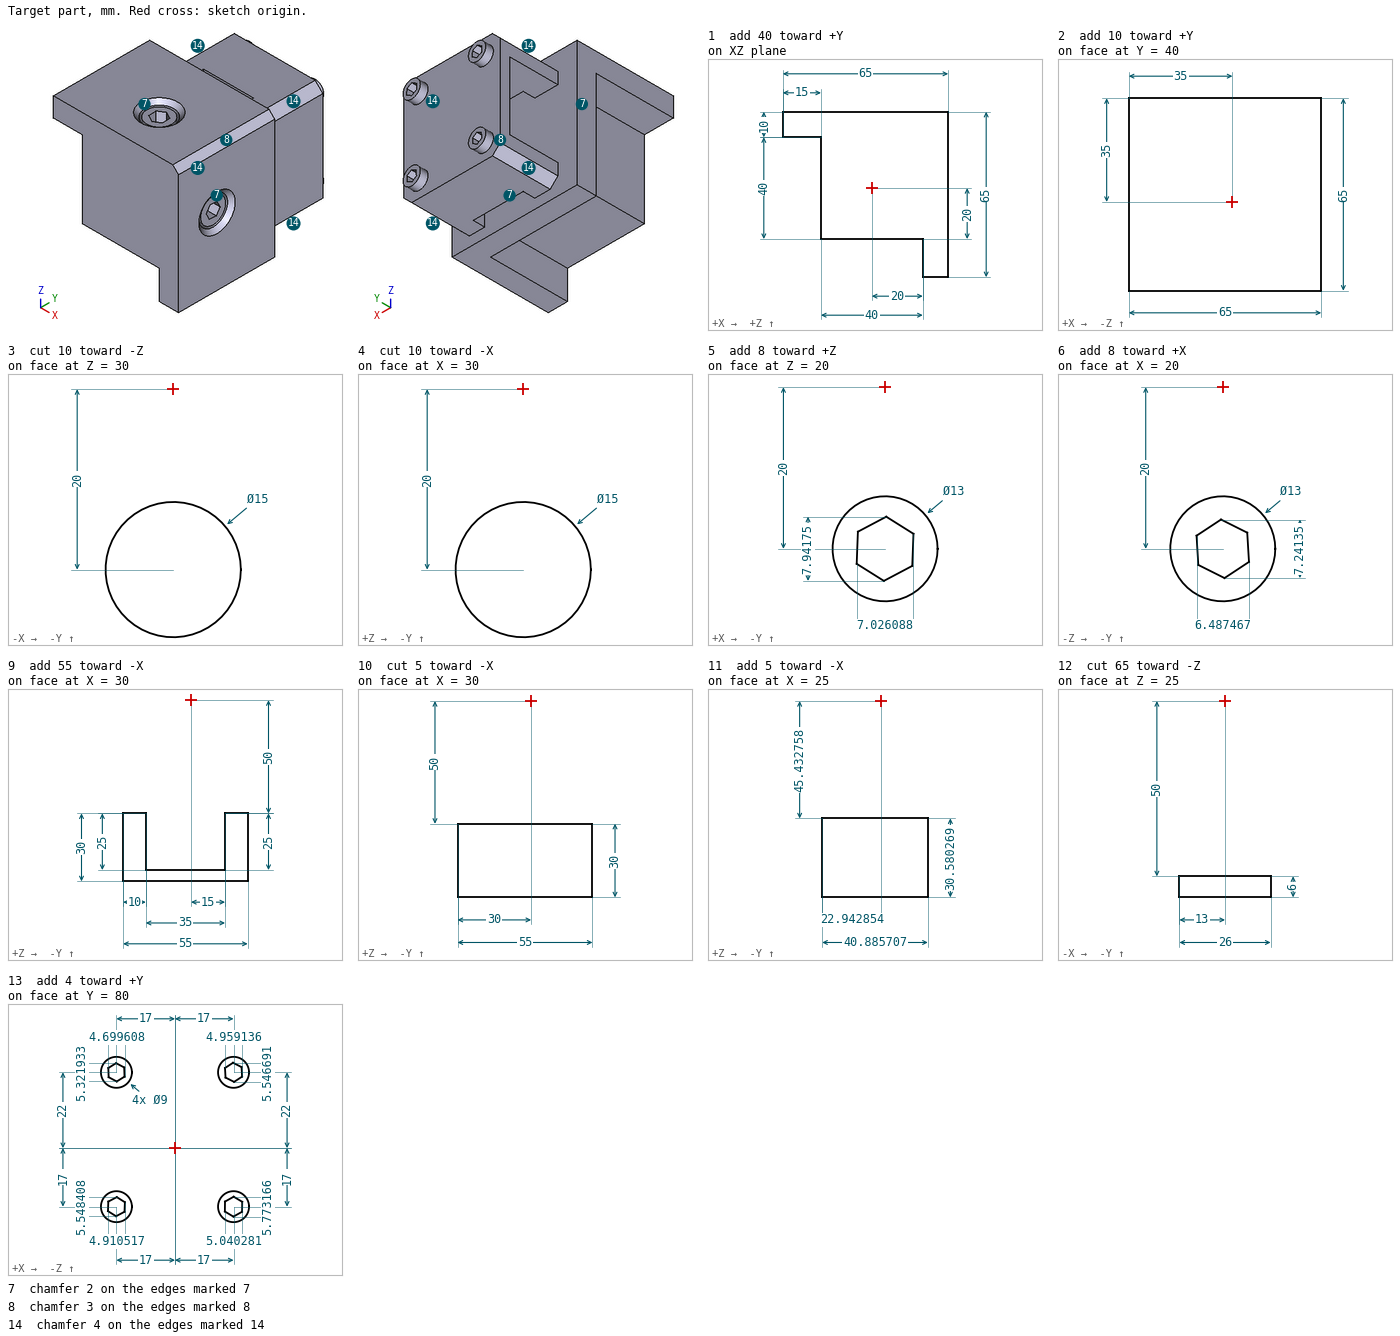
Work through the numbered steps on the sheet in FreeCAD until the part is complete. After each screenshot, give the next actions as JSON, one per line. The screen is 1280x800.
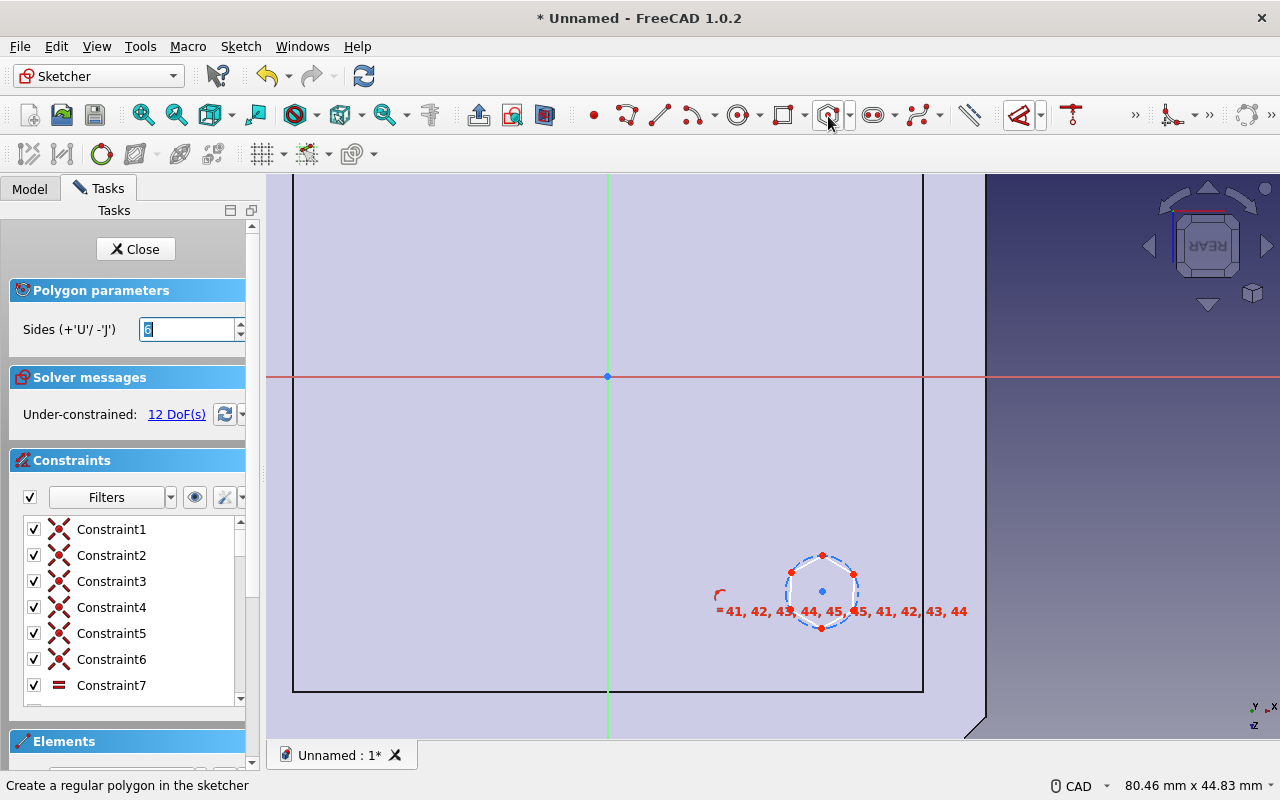
{"action": "left_click", "coordinate": [394, 591]}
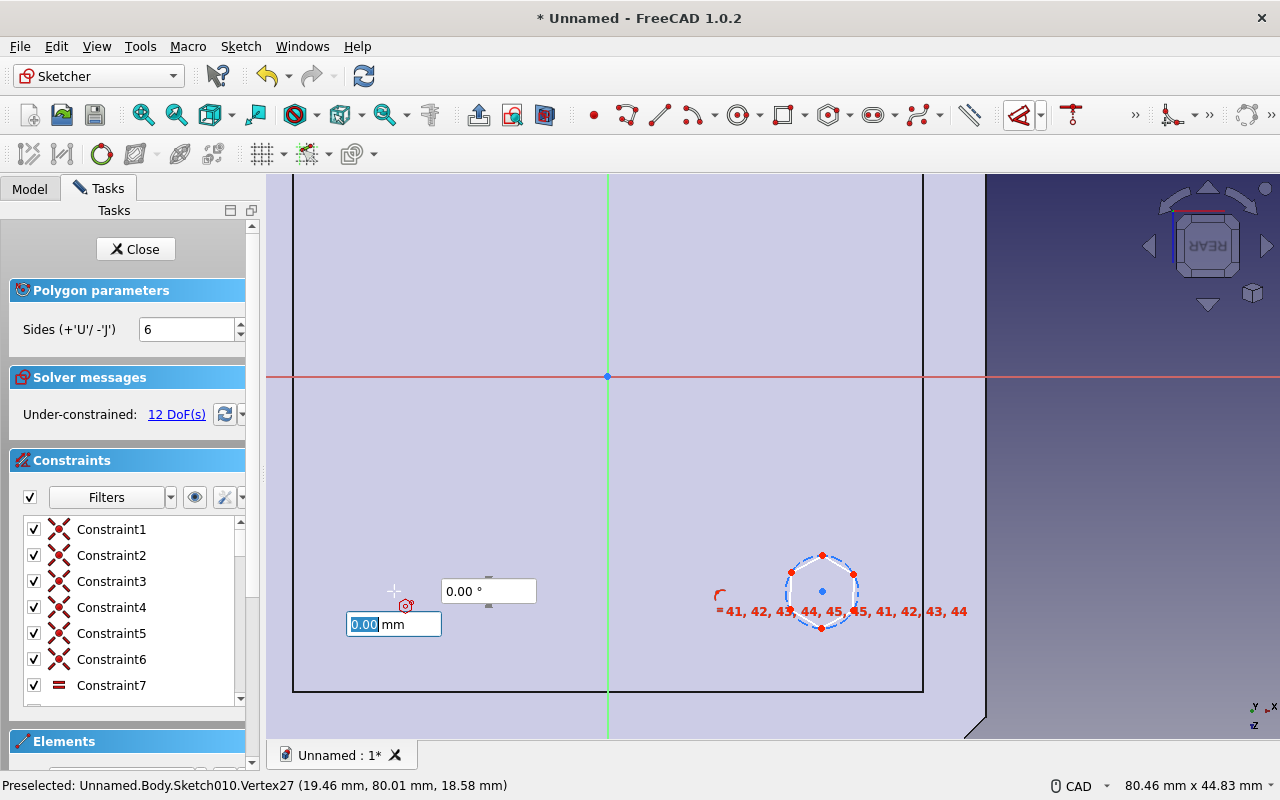
{"action": "left_click", "coordinate": [363, 607]}
{"action": "right_click", "coordinate": [363, 607]}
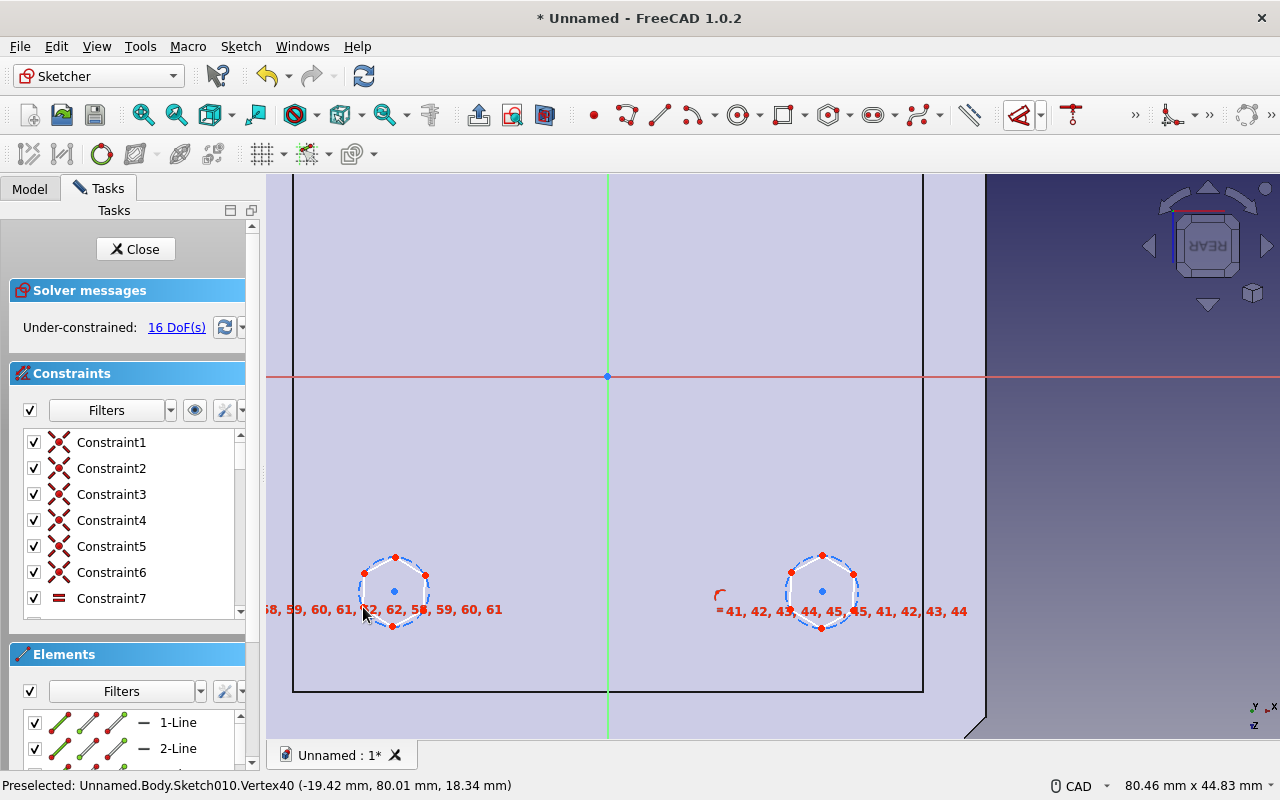
{"action": "left_click", "coordinate": [738, 116]}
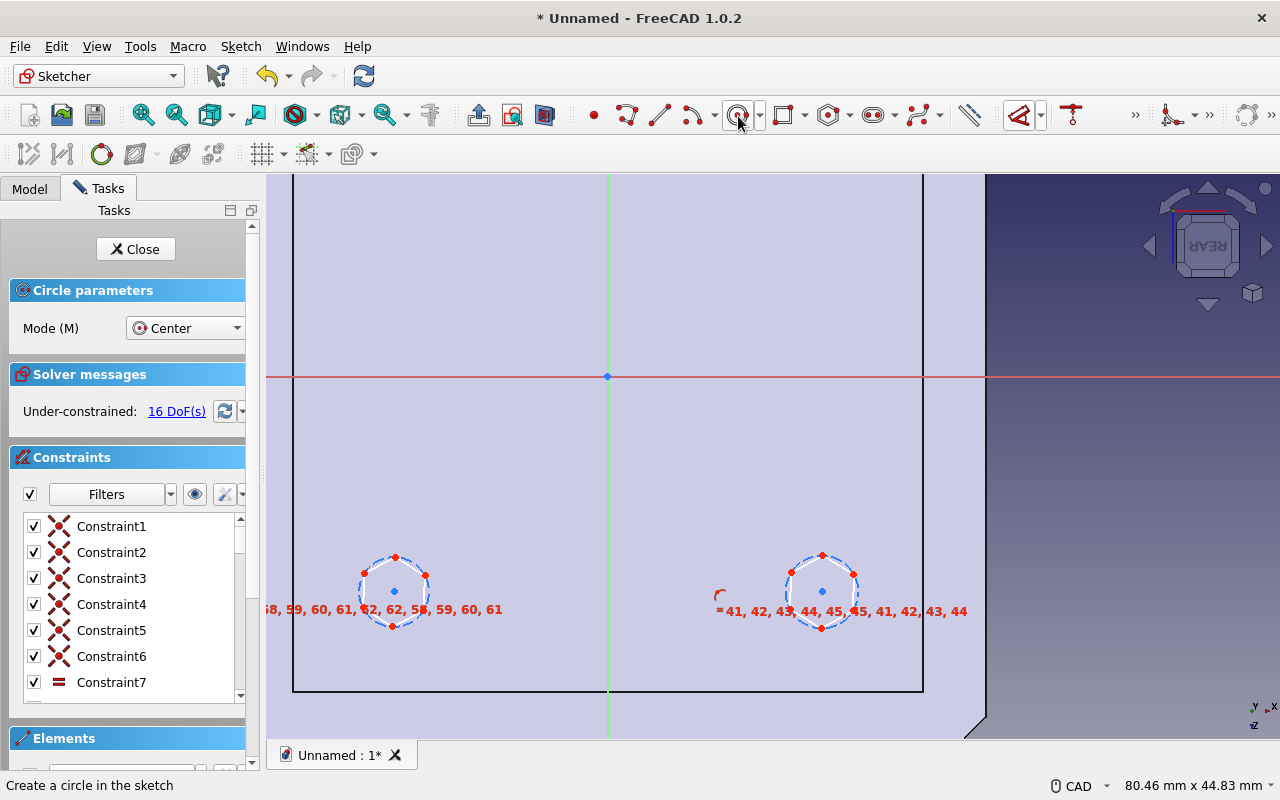
{"action": "scroll", "coordinate": [822, 592], "scroll_direction": "down", "scroll_amount": 3}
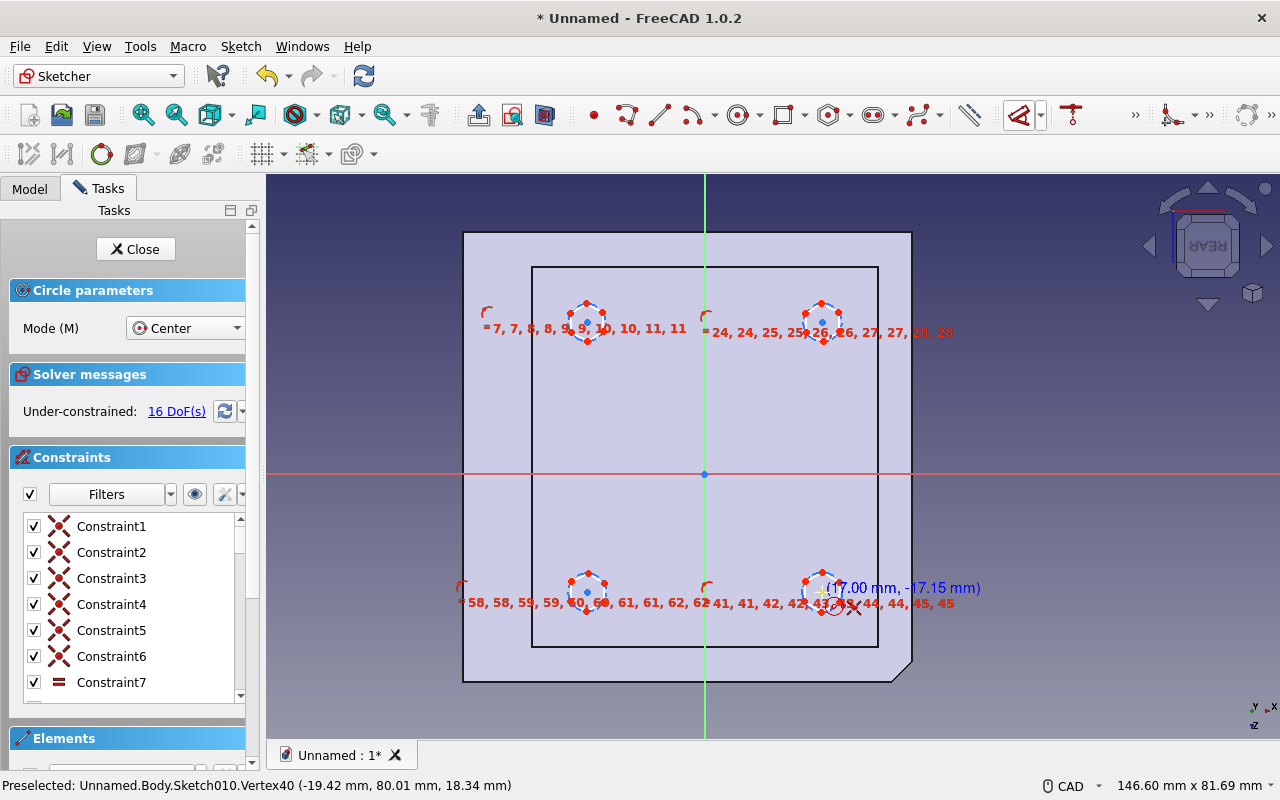
{"action": "left_click", "coordinate": [587, 323]}
{"action": "mouse_move", "coordinate": [565, 300]}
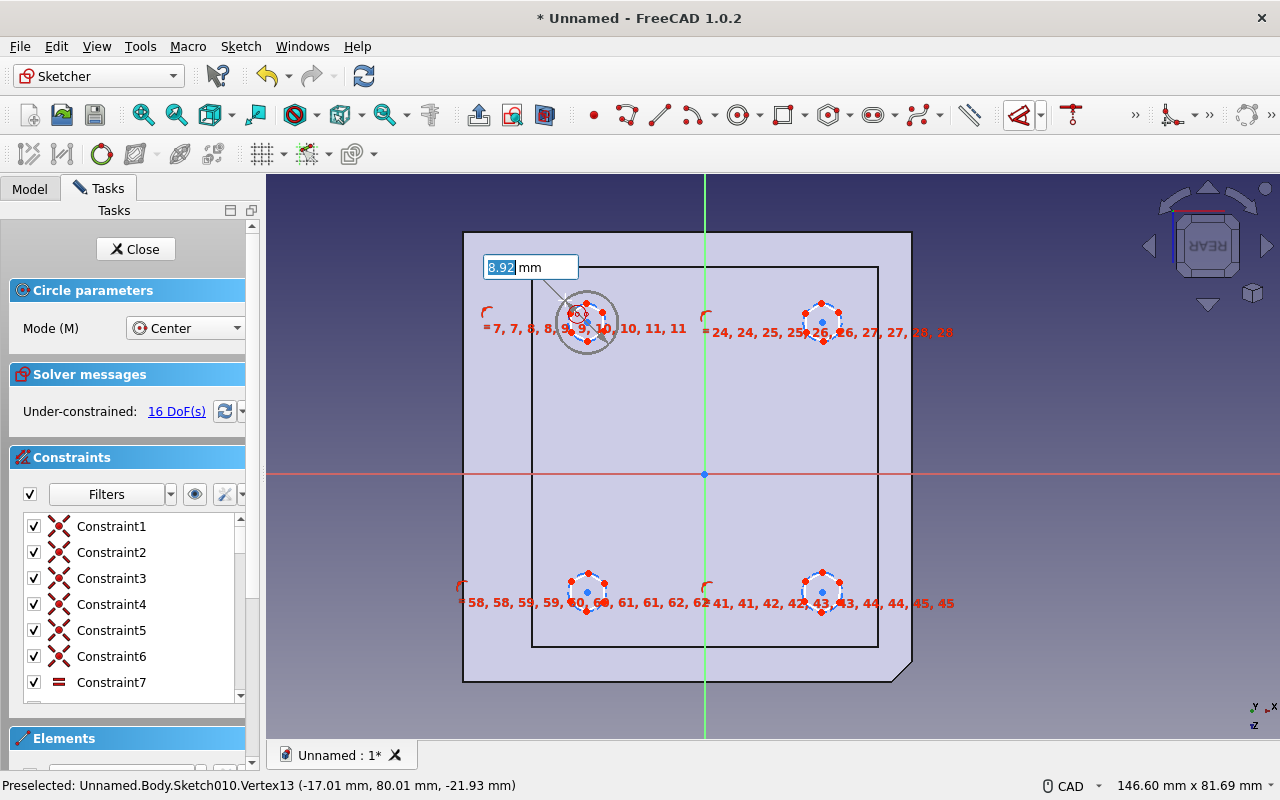
{"action": "type", "text": "9"}
{"action": "key", "text": "Return"}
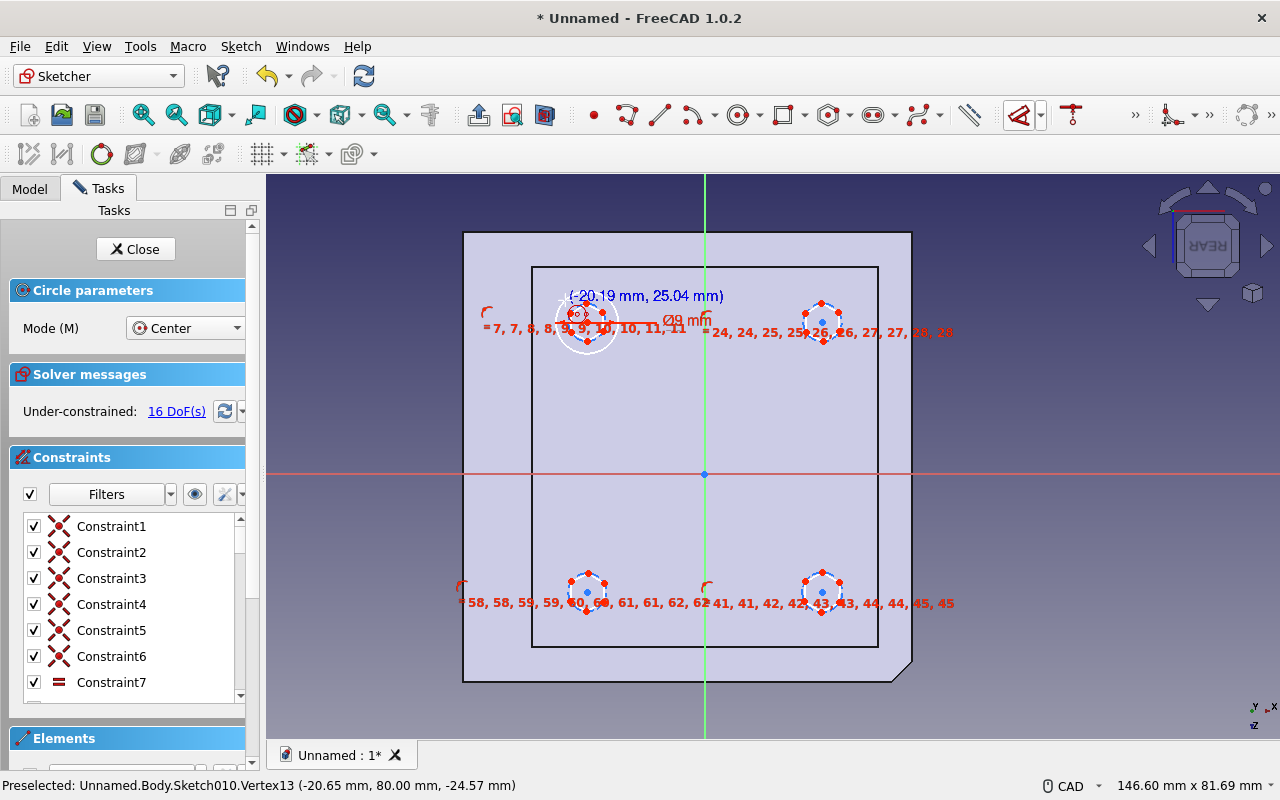
{"action": "left_click", "coordinate": [822, 323]}
{"action": "mouse_move", "coordinate": [833, 293]}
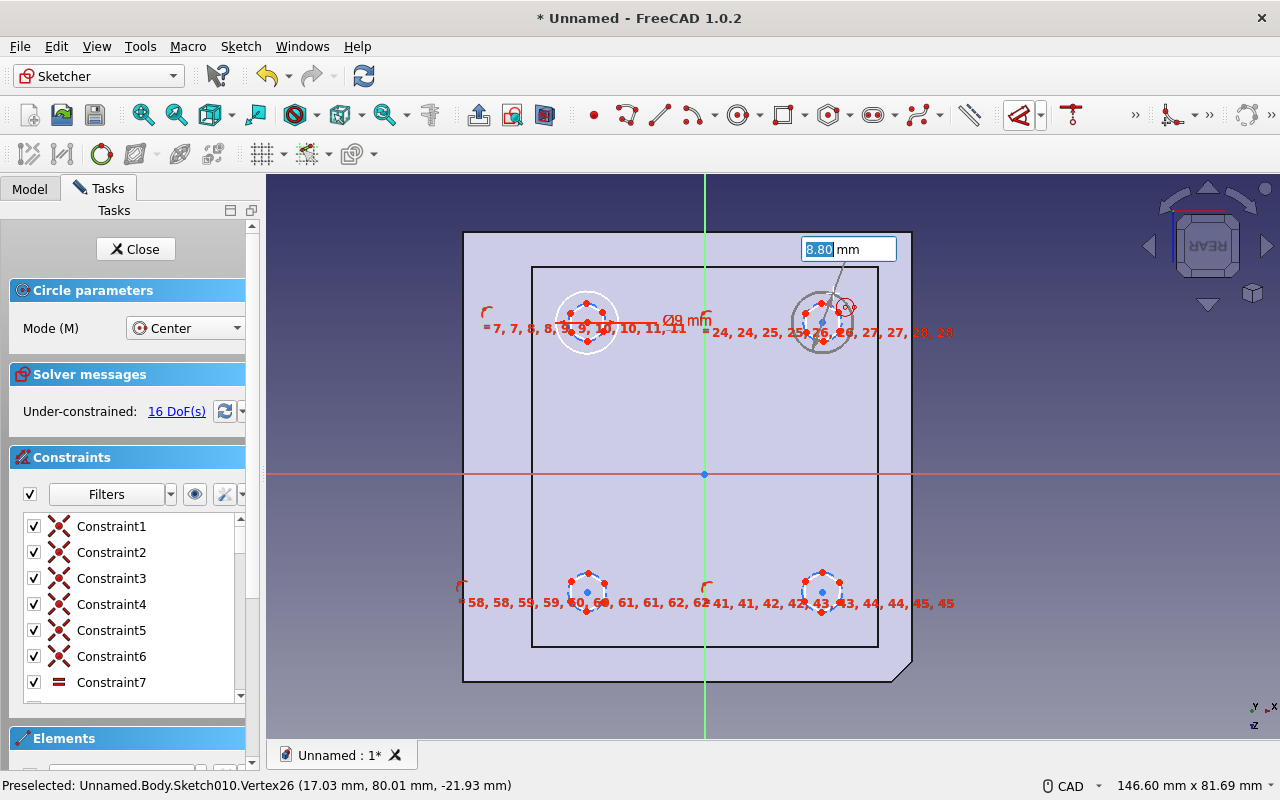
{"action": "type", "text": "9"}
{"action": "key", "text": "Return"}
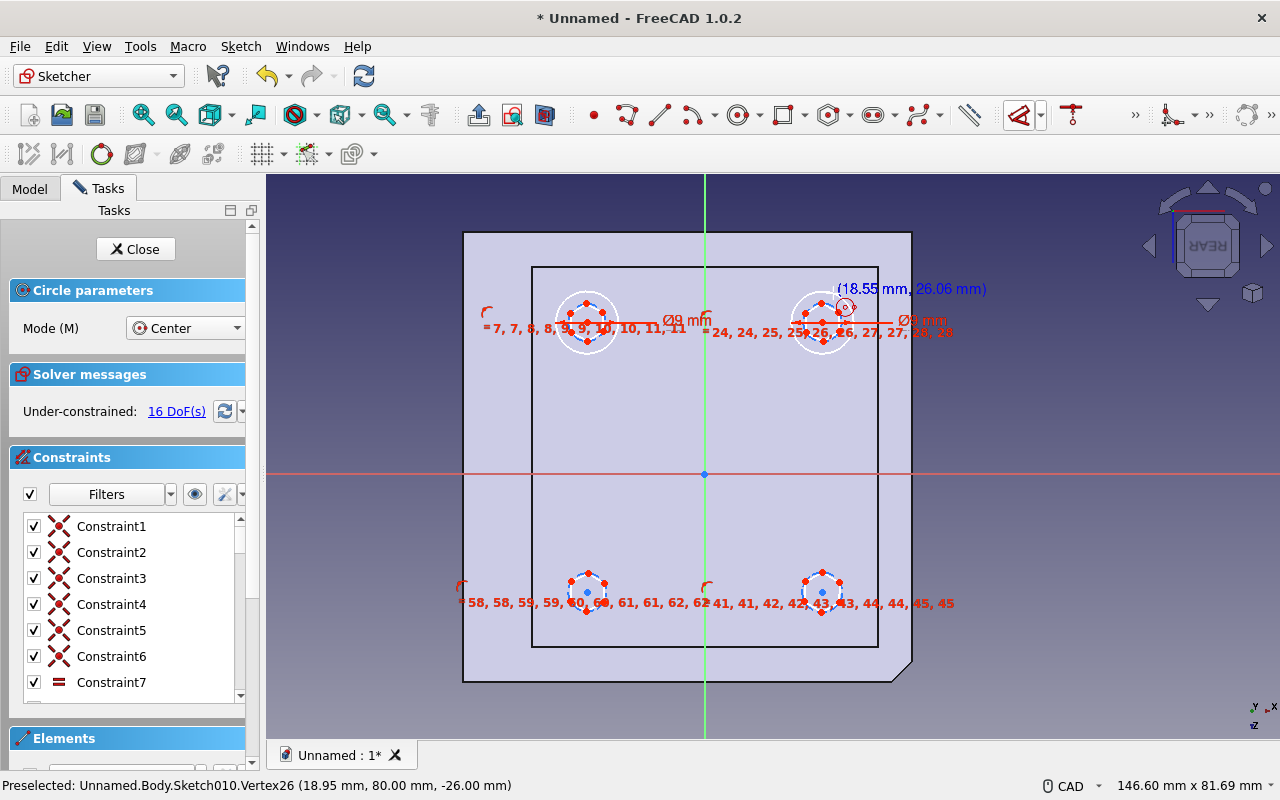
{"action": "left_click", "coordinate": [822, 592]}
{"action": "mouse_move", "coordinate": [833, 563]}